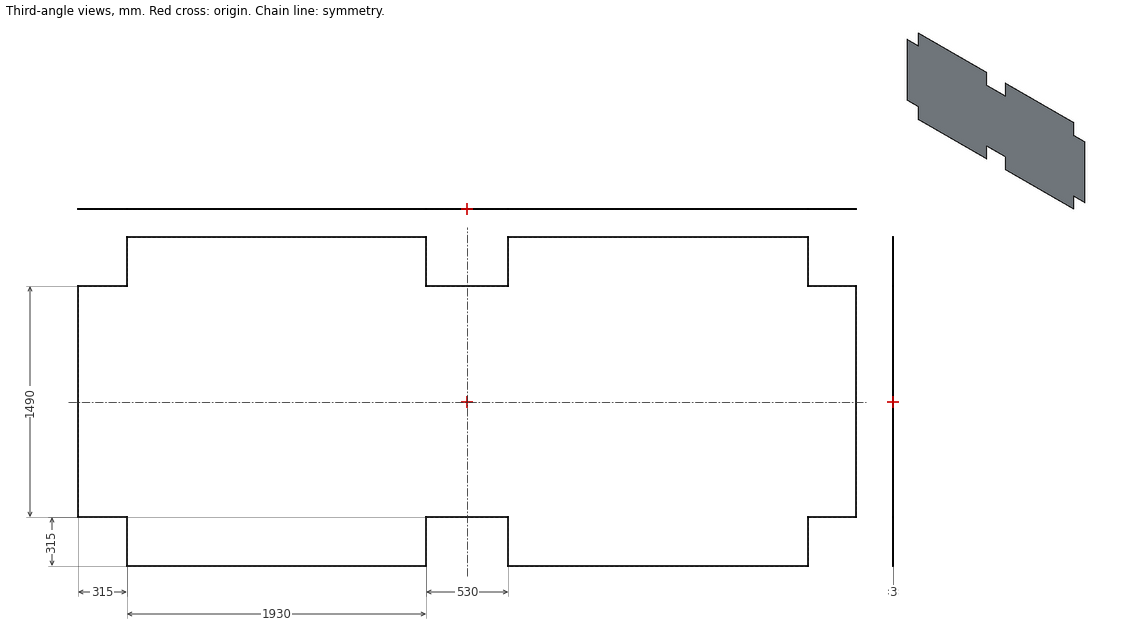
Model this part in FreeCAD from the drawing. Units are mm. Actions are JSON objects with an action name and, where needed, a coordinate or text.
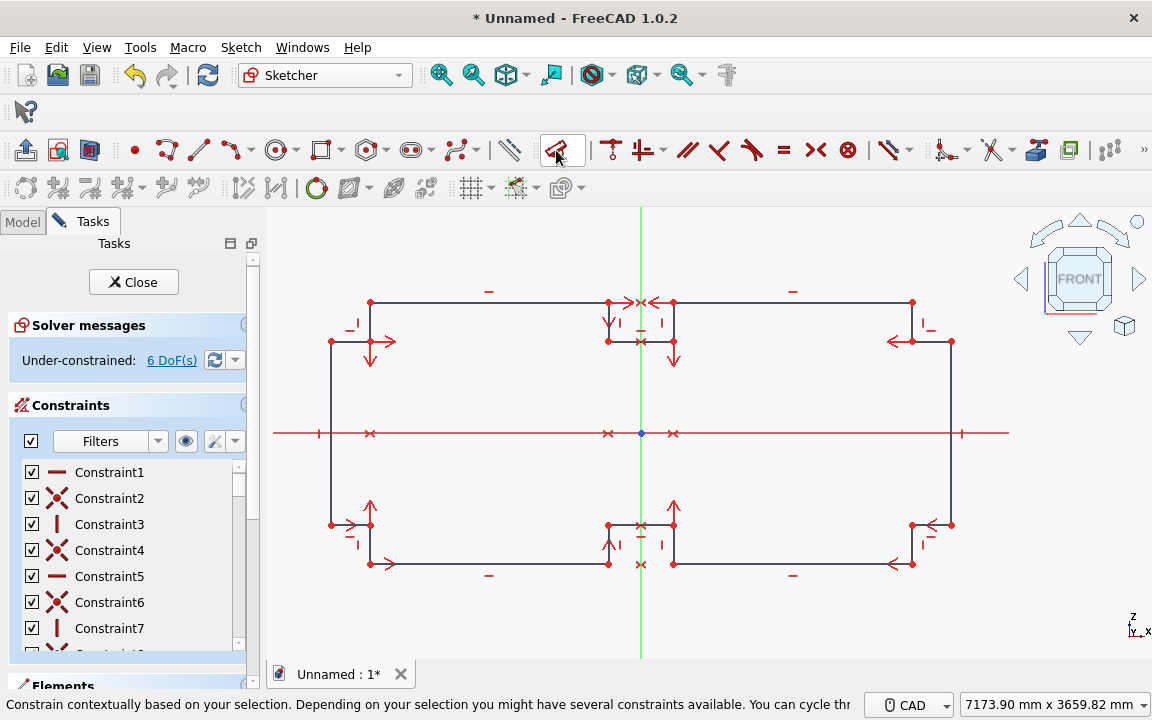
{"action": "left_click", "coordinate": [654, 525]}
{"action": "left_click", "coordinate": [626, 559]}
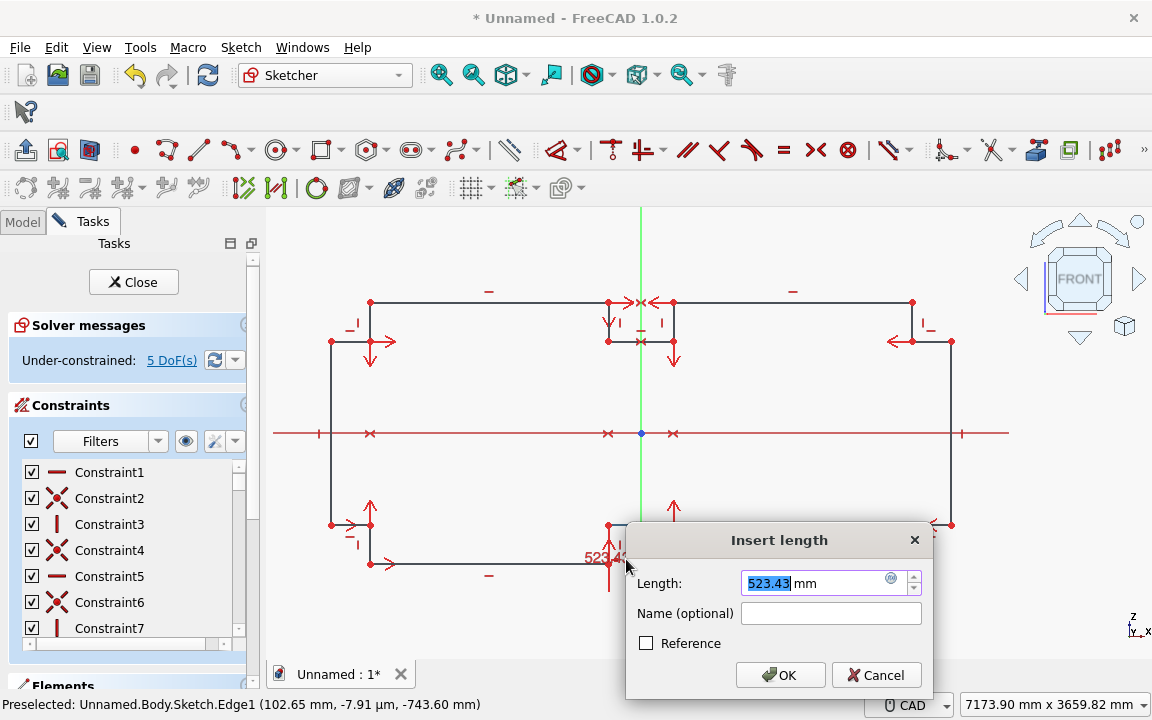
{"action": "type", "text": "530"}
{"action": "key", "text": "Return"}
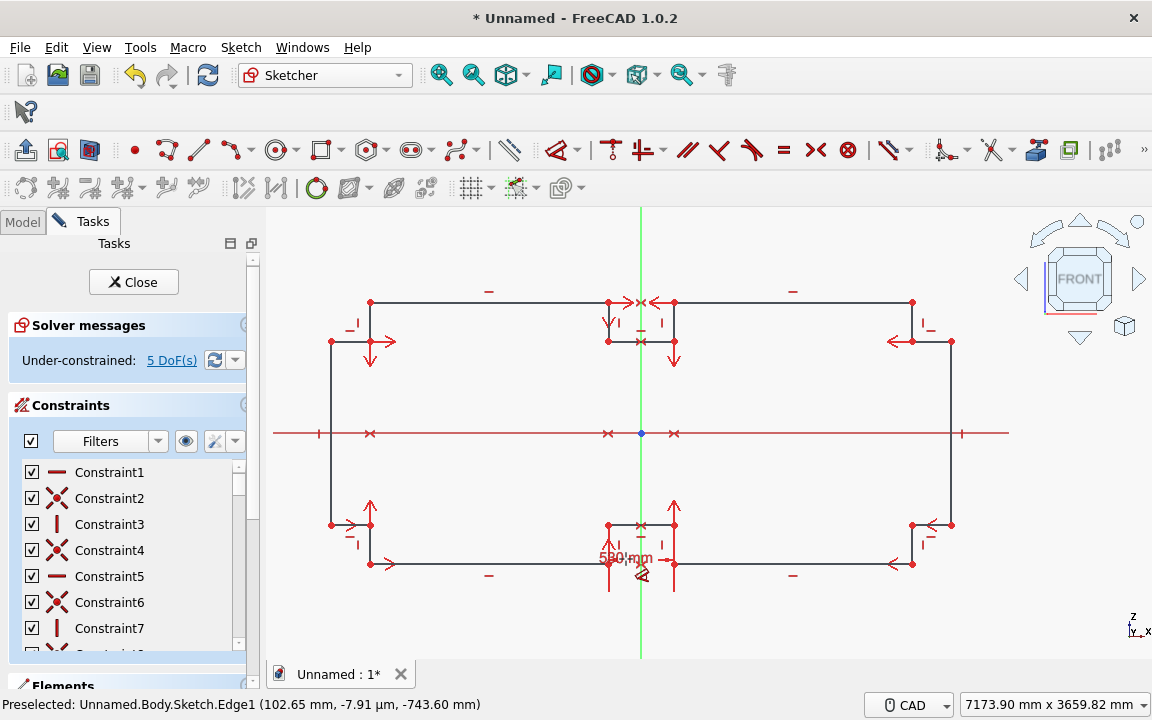
{"action": "left_click", "coordinate": [609, 537]}
{"action": "left_click", "coordinate": [575, 536]}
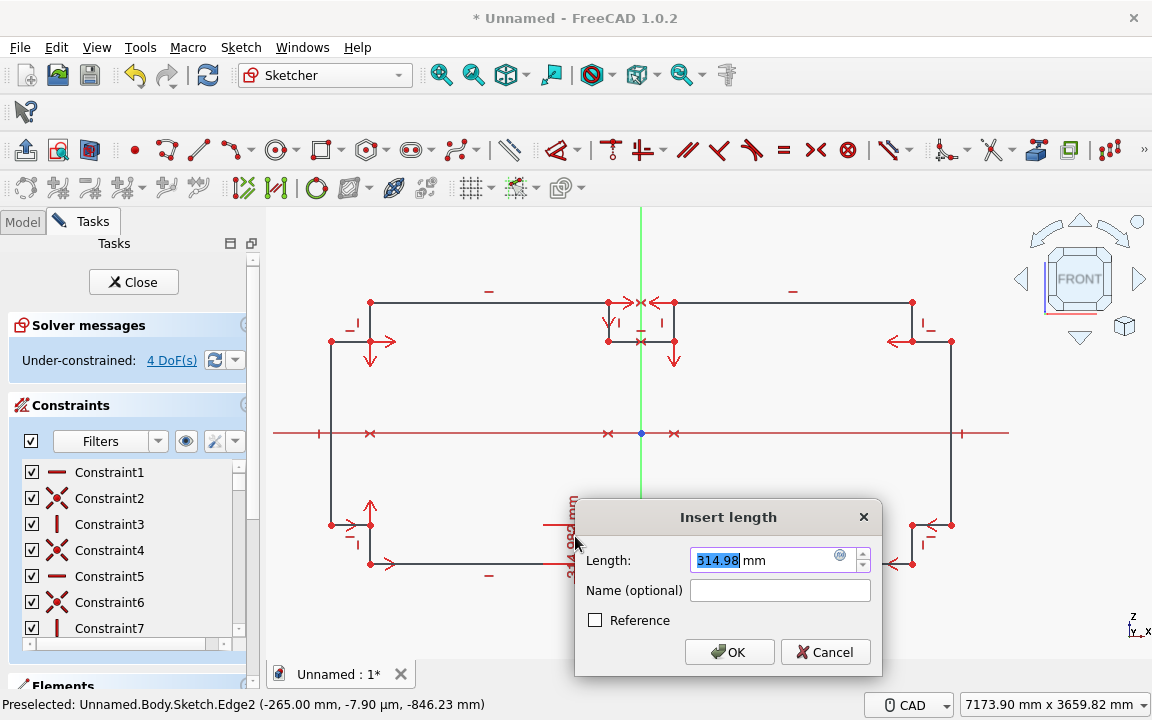
{"action": "type", "text": "315"}
{"action": "key", "text": "Return"}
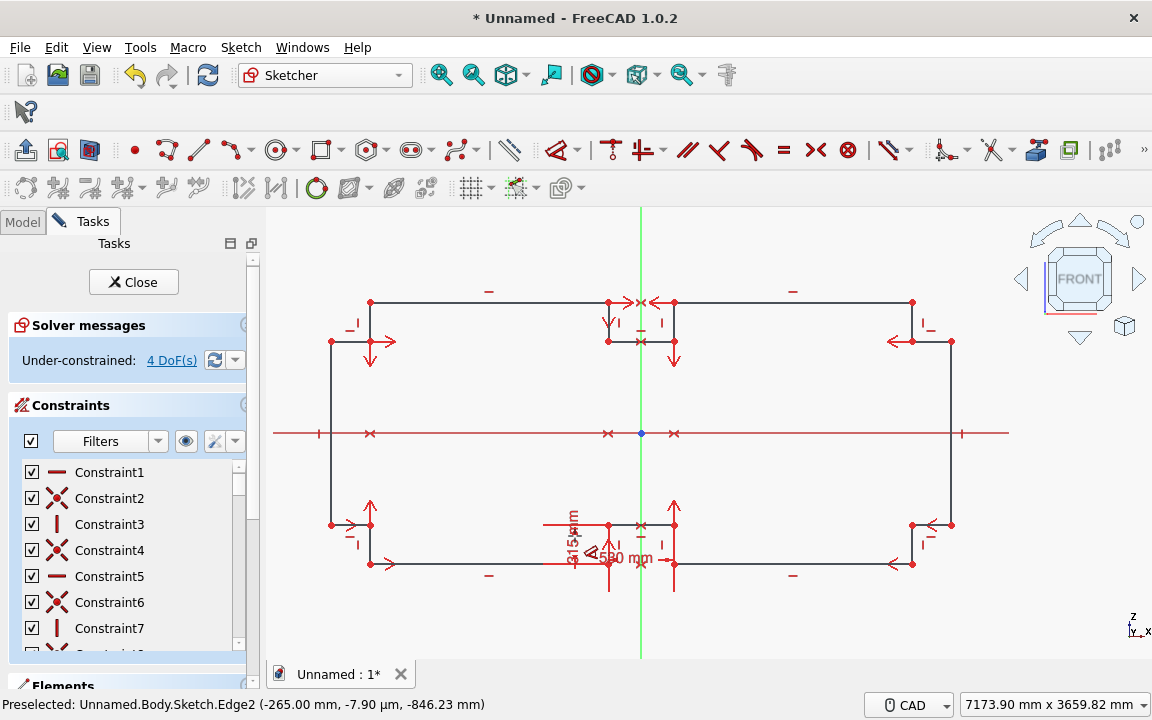
{"action": "left_click", "coordinate": [370, 553]}
{"action": "left_click", "coordinate": [336, 545]}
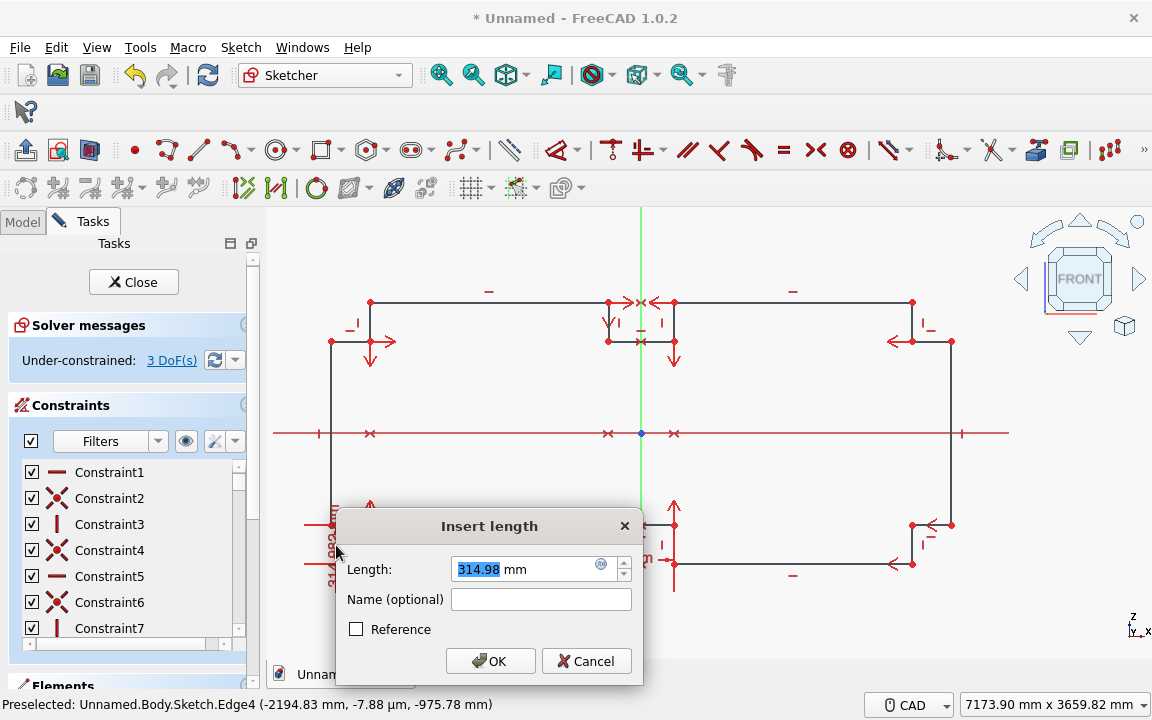
{"action": "type", "text": "315"}
{"action": "key", "text": "Return"}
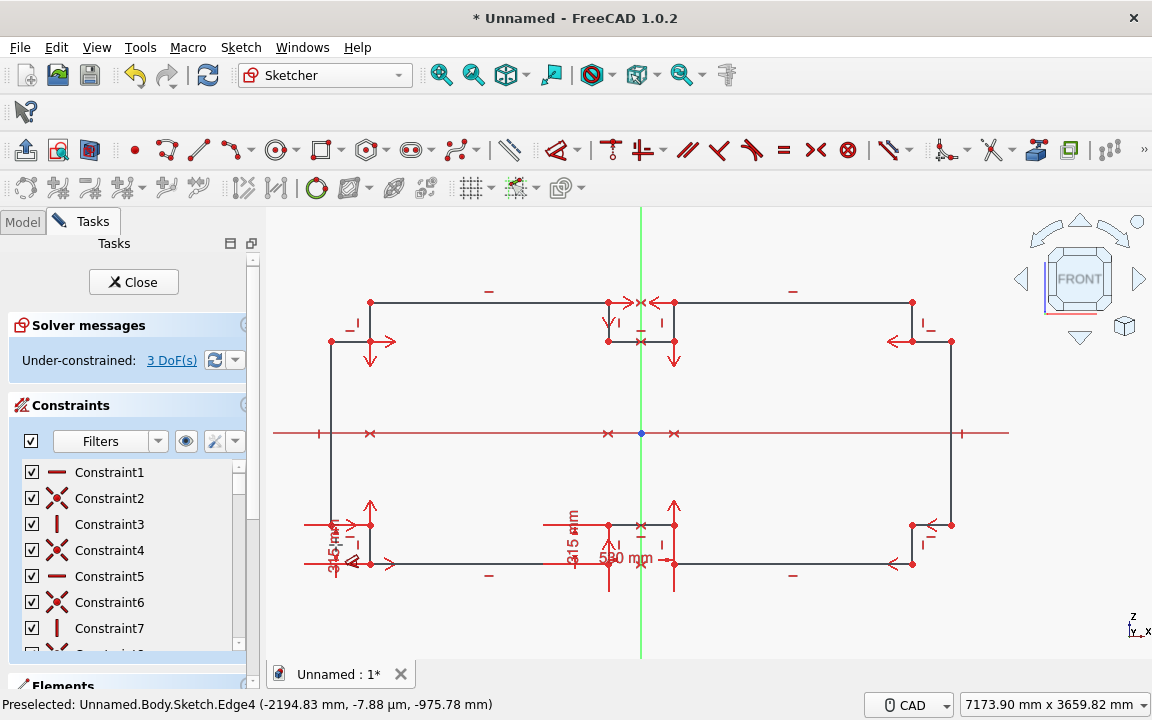
{"action": "left_click", "coordinate": [359, 525]}
{"action": "left_click", "coordinate": [351, 491]}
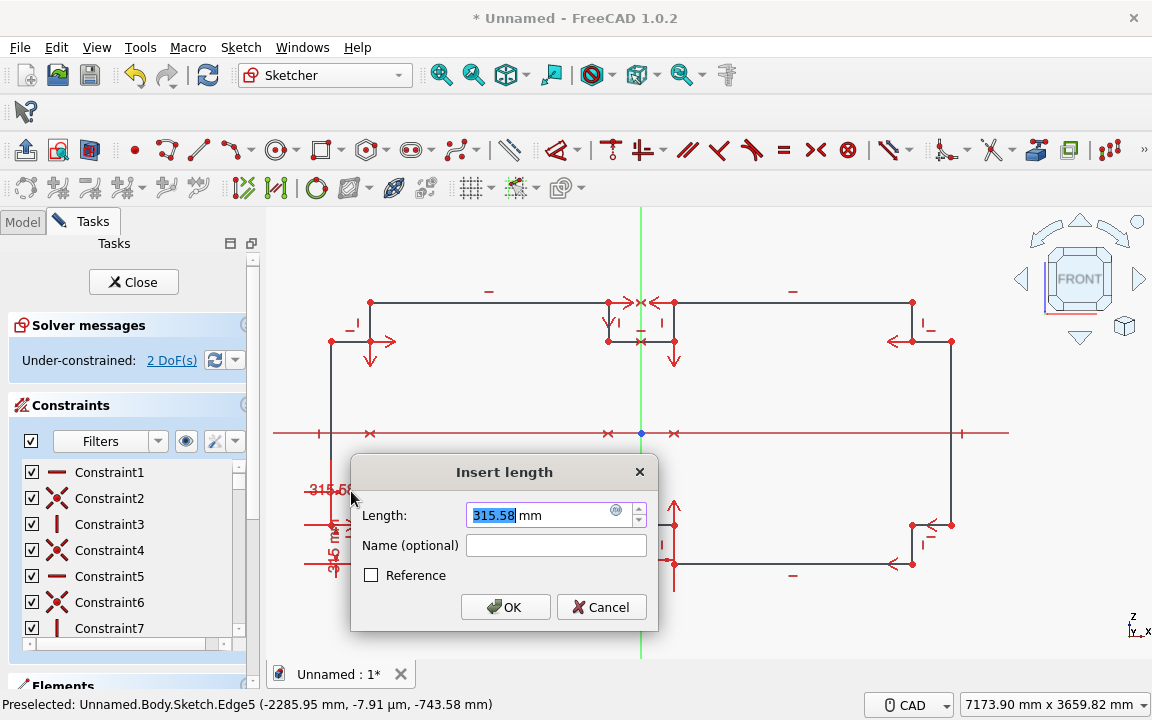
{"action": "type", "text": "315"}
{"action": "key", "text": "Return"}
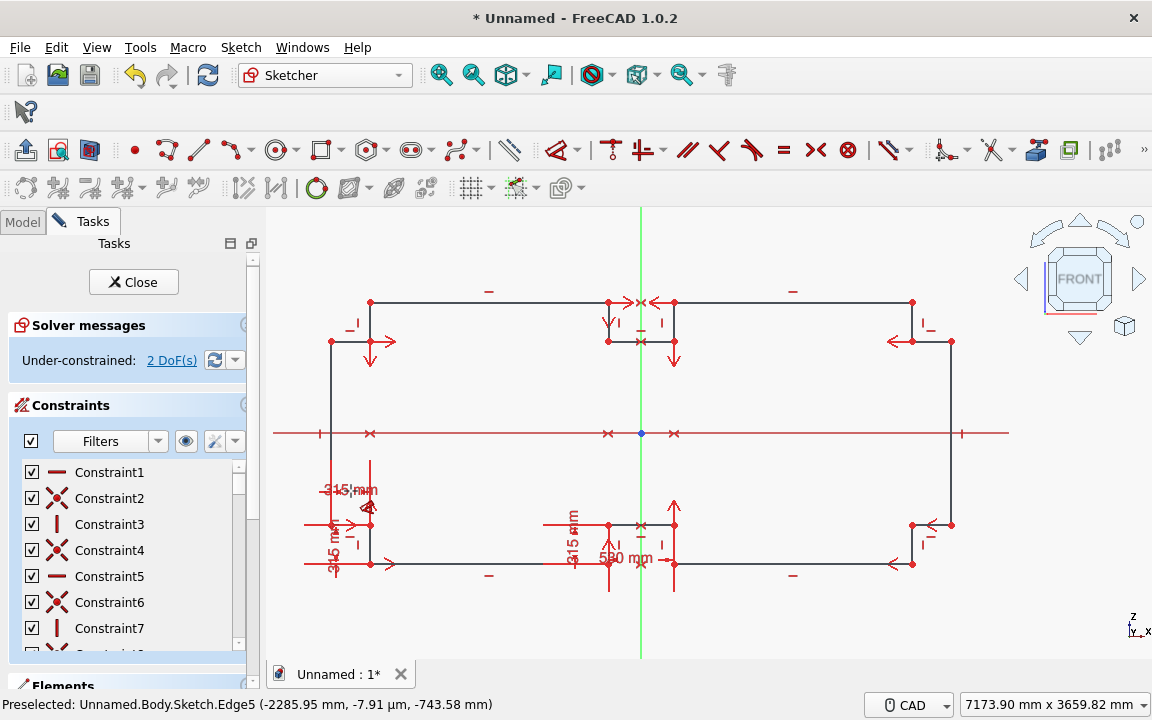
{"action": "left_click", "coordinate": [537, 564]}
{"action": "left_click", "coordinate": [489, 598]}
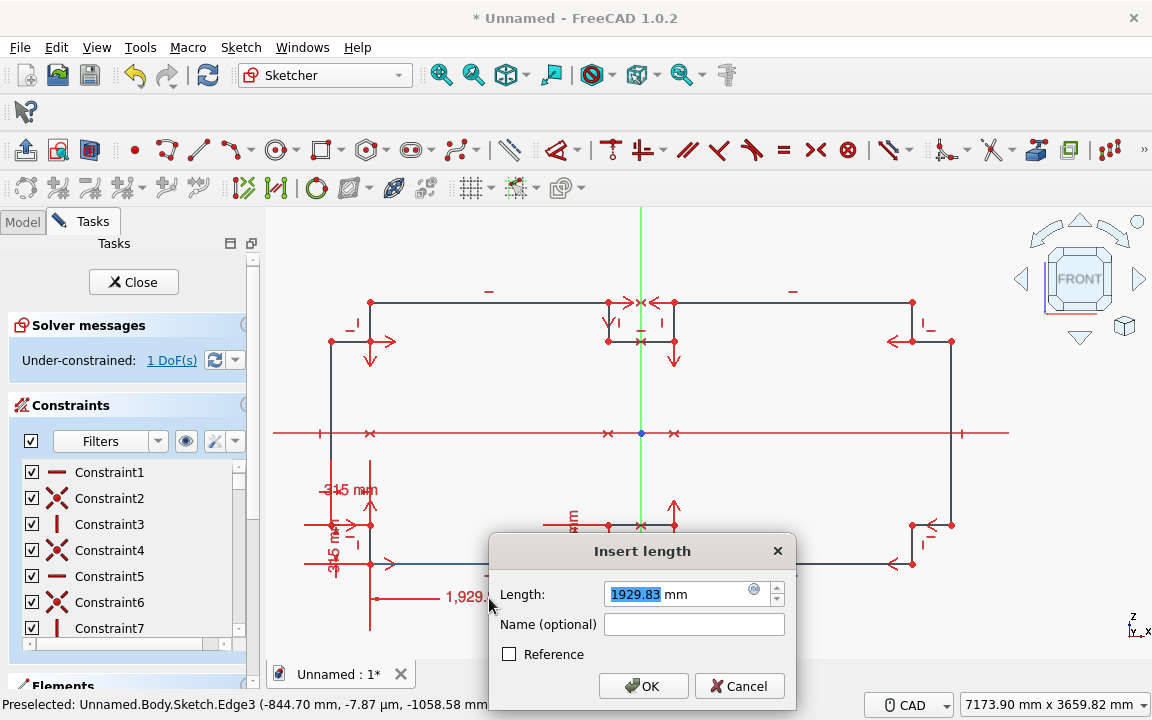
{"action": "type", "text": "1930"}
{"action": "key", "text": "Return"}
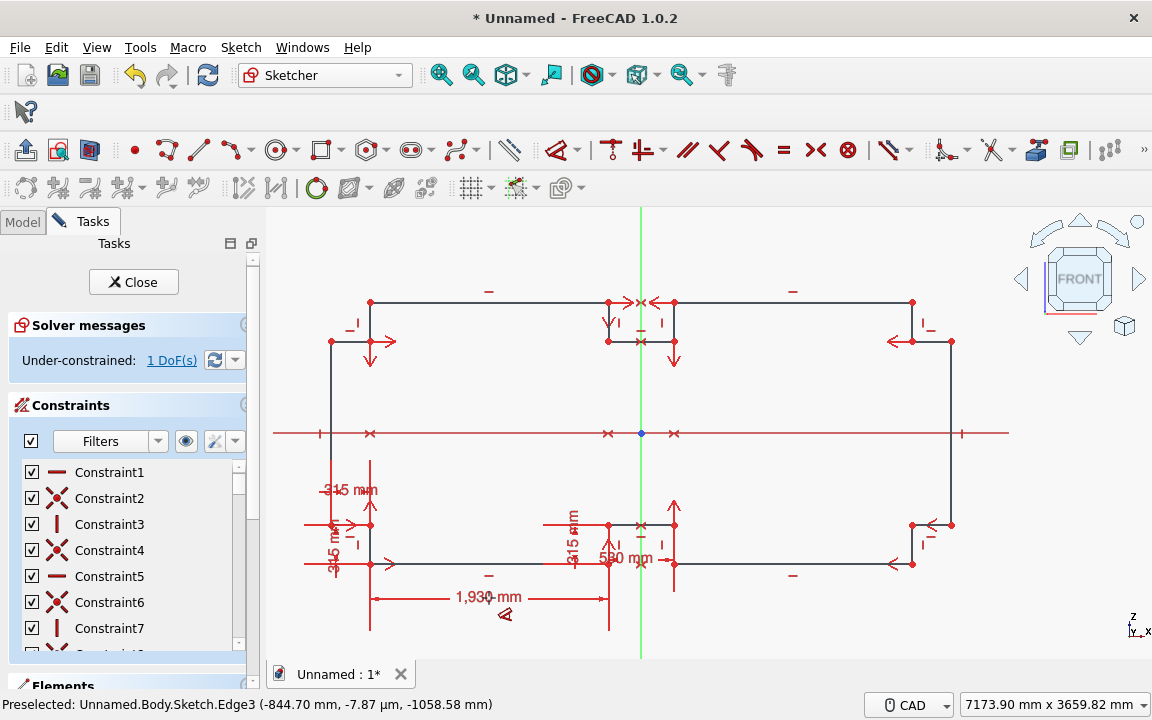
{"action": "left_click", "coordinate": [331, 470]}
{"action": "left_click", "coordinate": [297, 391]}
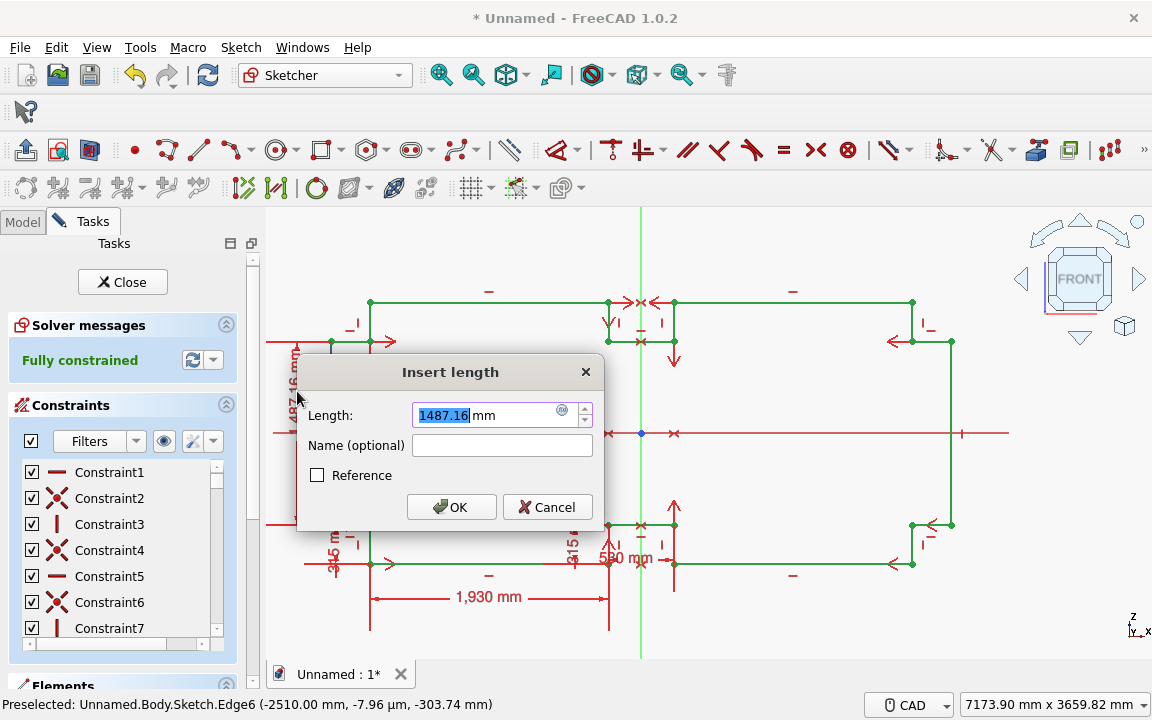
{"action": "type", "text": "1490"}
{"action": "key", "text": "Return"}
{"action": "key", "text": "Escape"}